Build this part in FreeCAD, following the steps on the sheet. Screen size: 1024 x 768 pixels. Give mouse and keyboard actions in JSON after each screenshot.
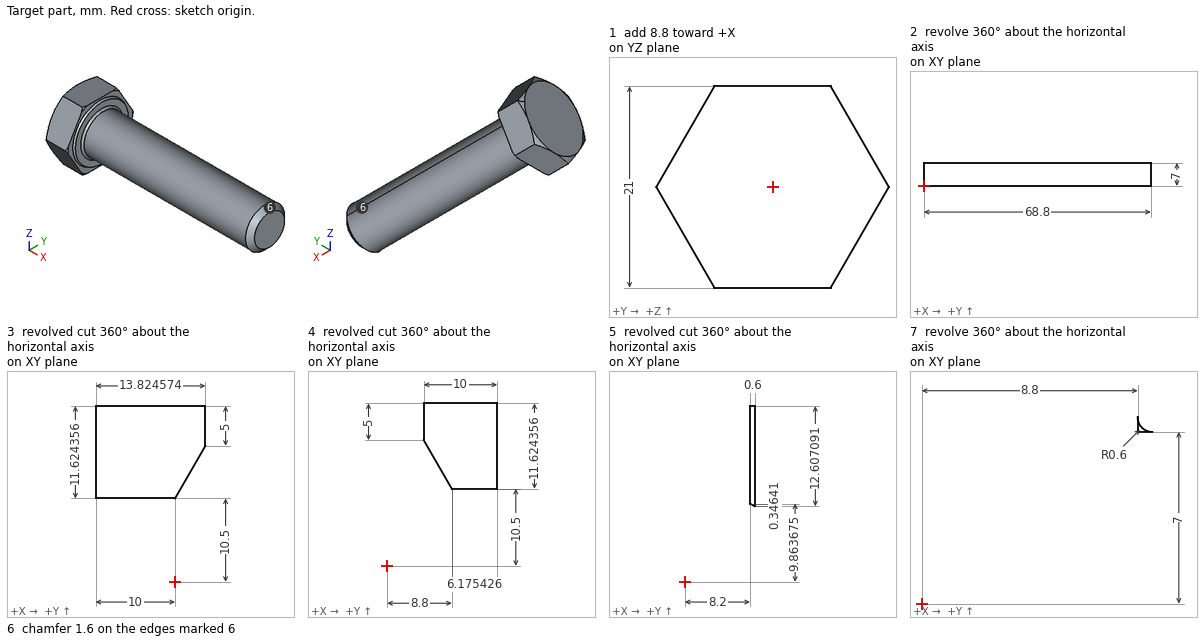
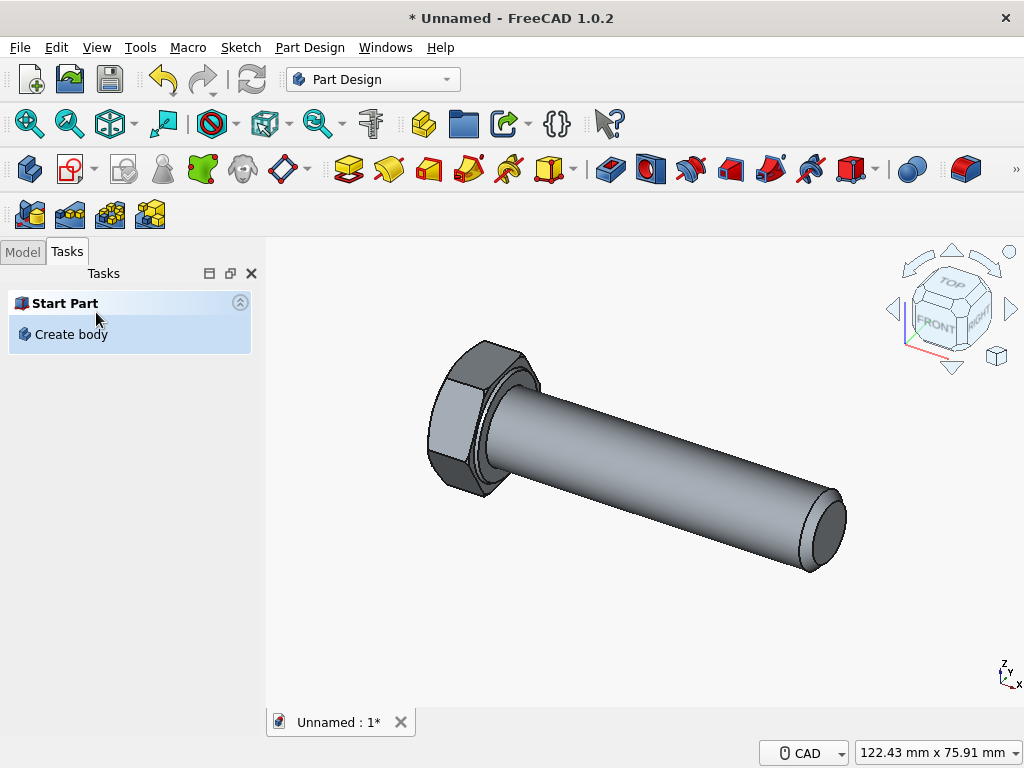
{"action": "left_click", "coordinate": [70, 170]}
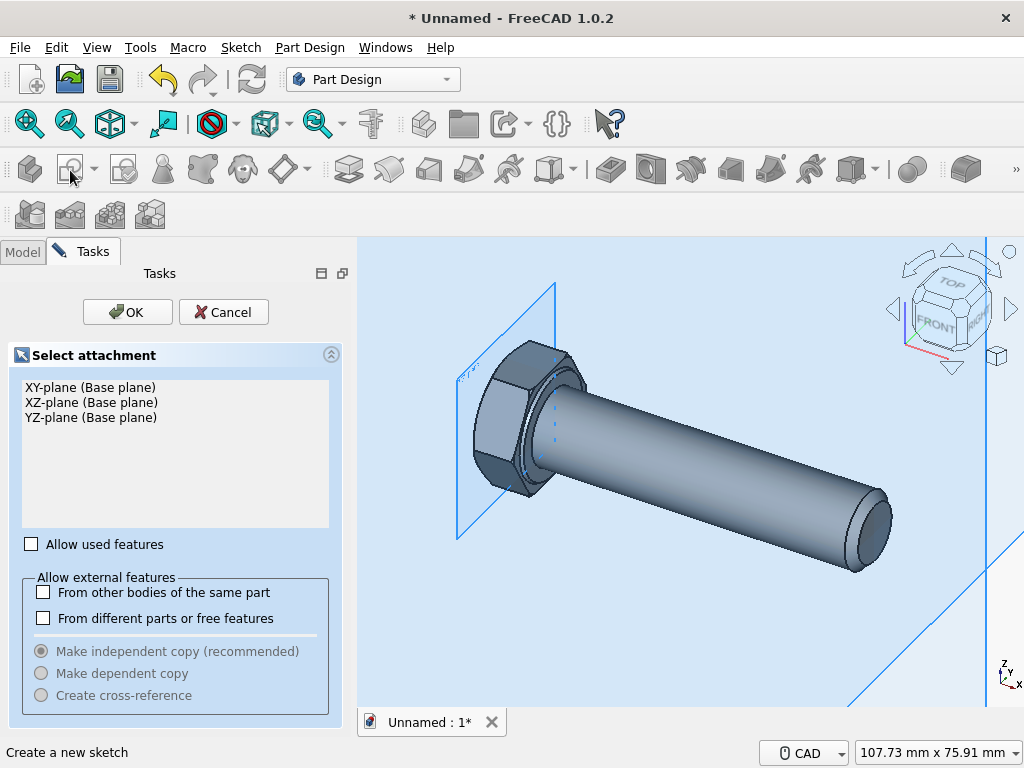
{"action": "left_click", "coordinate": [82, 388]}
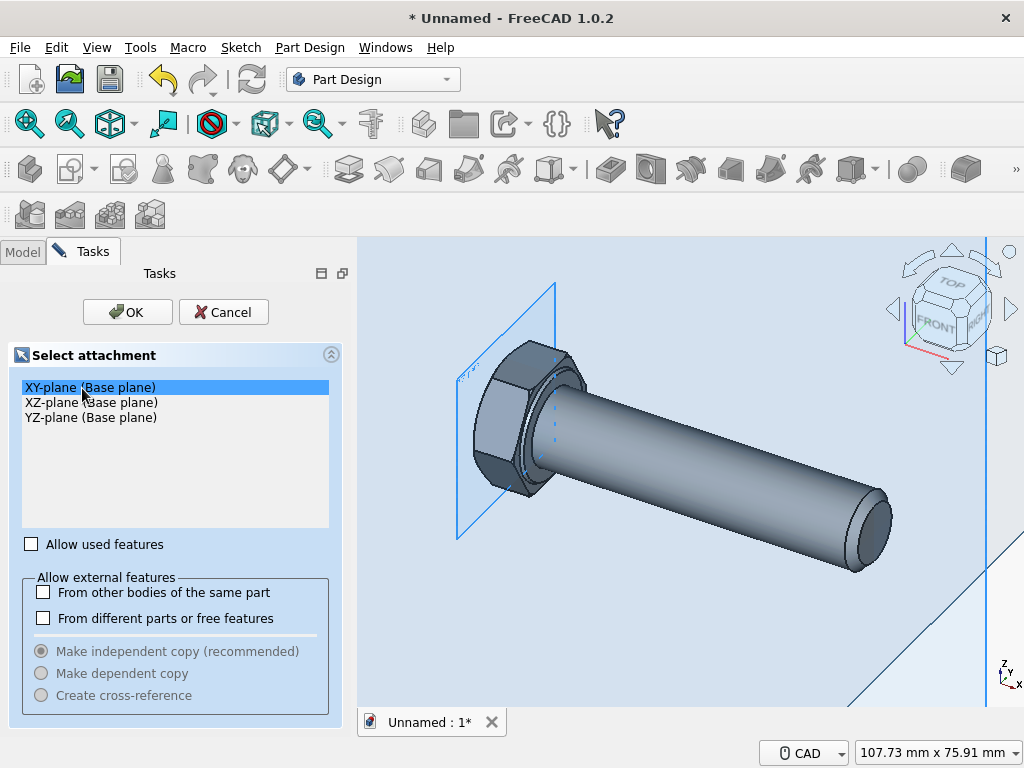
{"action": "left_click", "coordinate": [128, 312]}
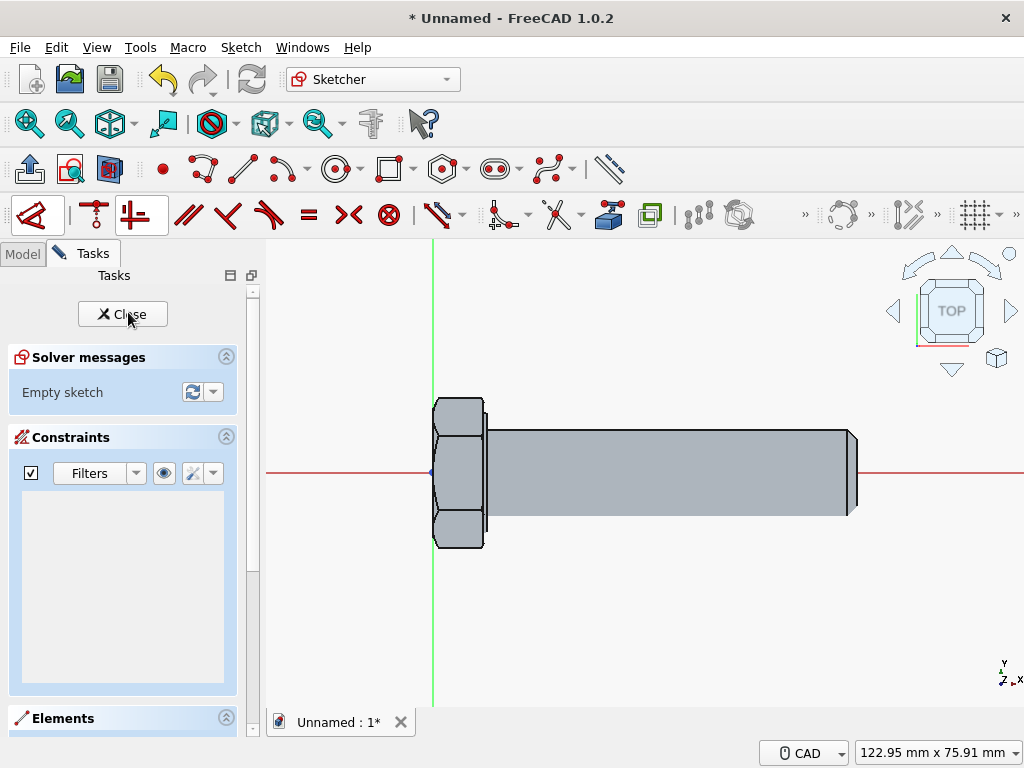
{"action": "left_click", "coordinate": [110, 170]}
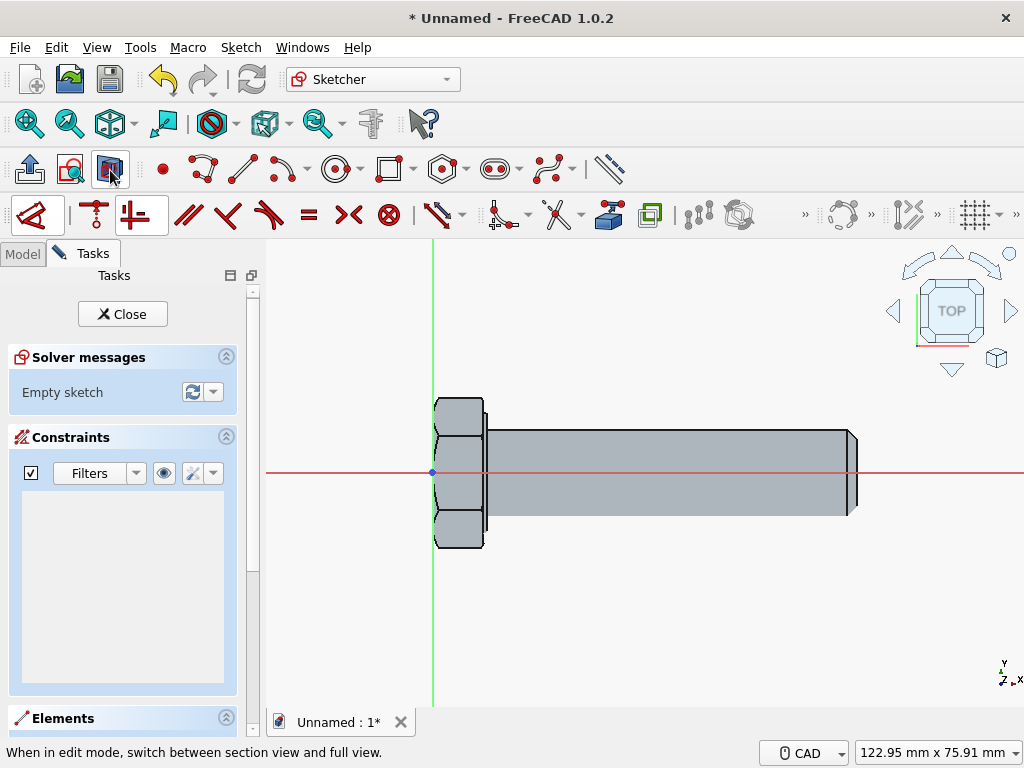
{"action": "scroll", "coordinate": [484, 426], "scroll_direction": "up", "scroll_amount": 15}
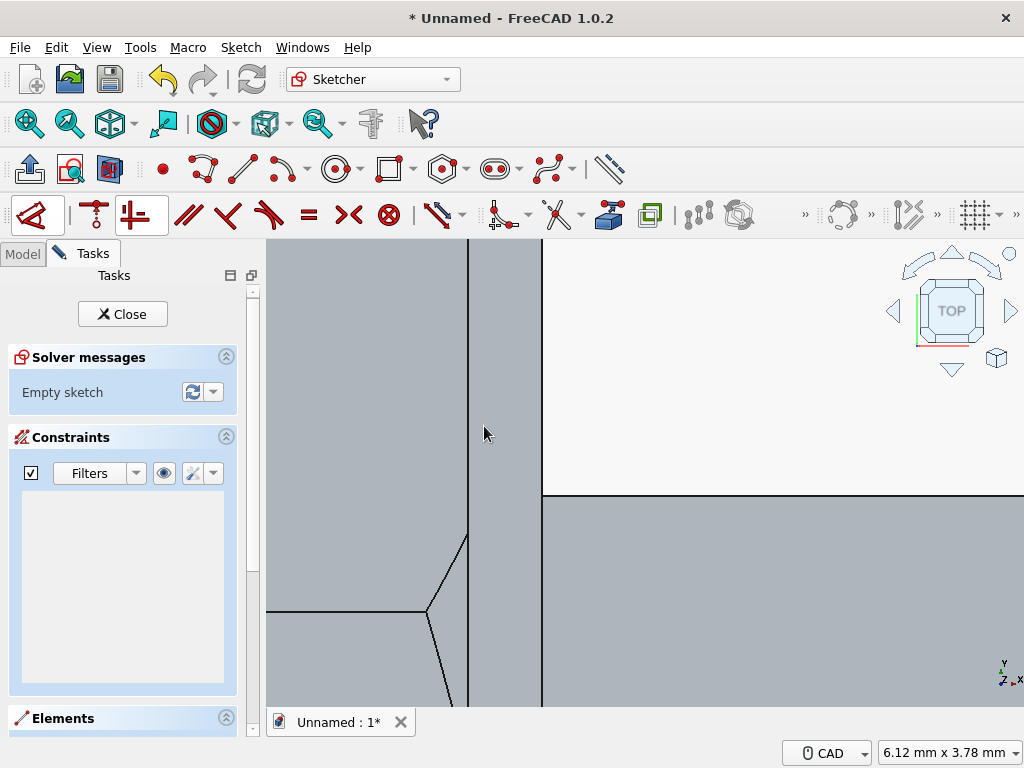
{"action": "scroll", "coordinate": [580, 454], "scroll_direction": "up", "scroll_amount": 7}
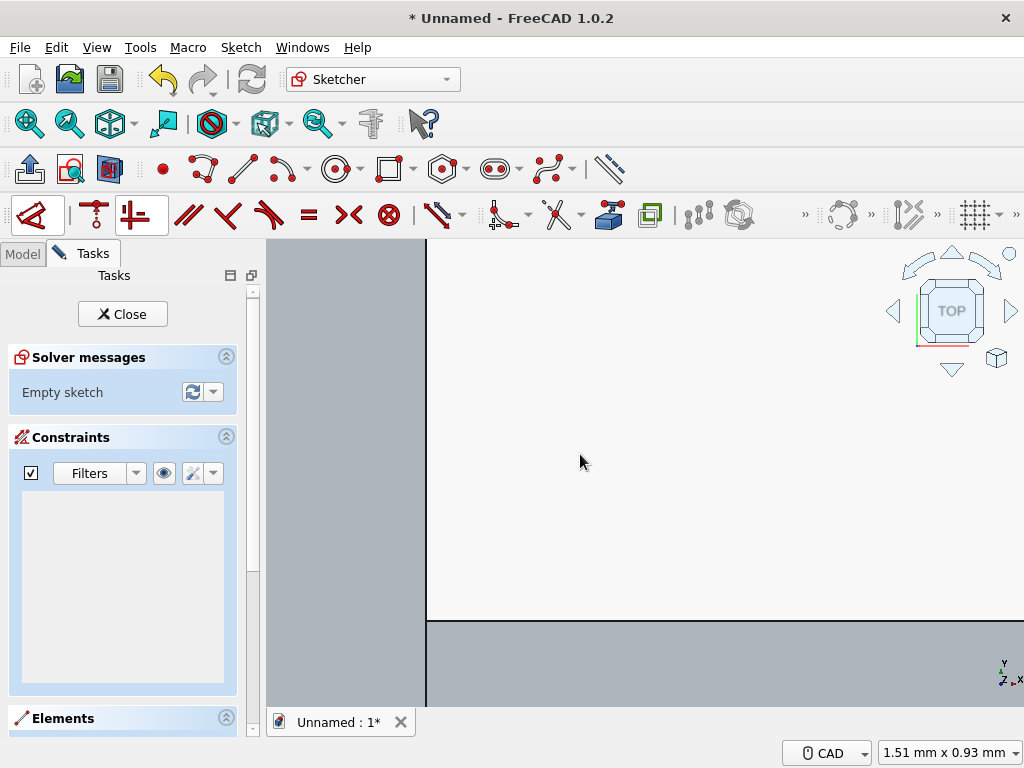
{"action": "key", "text": "g m"}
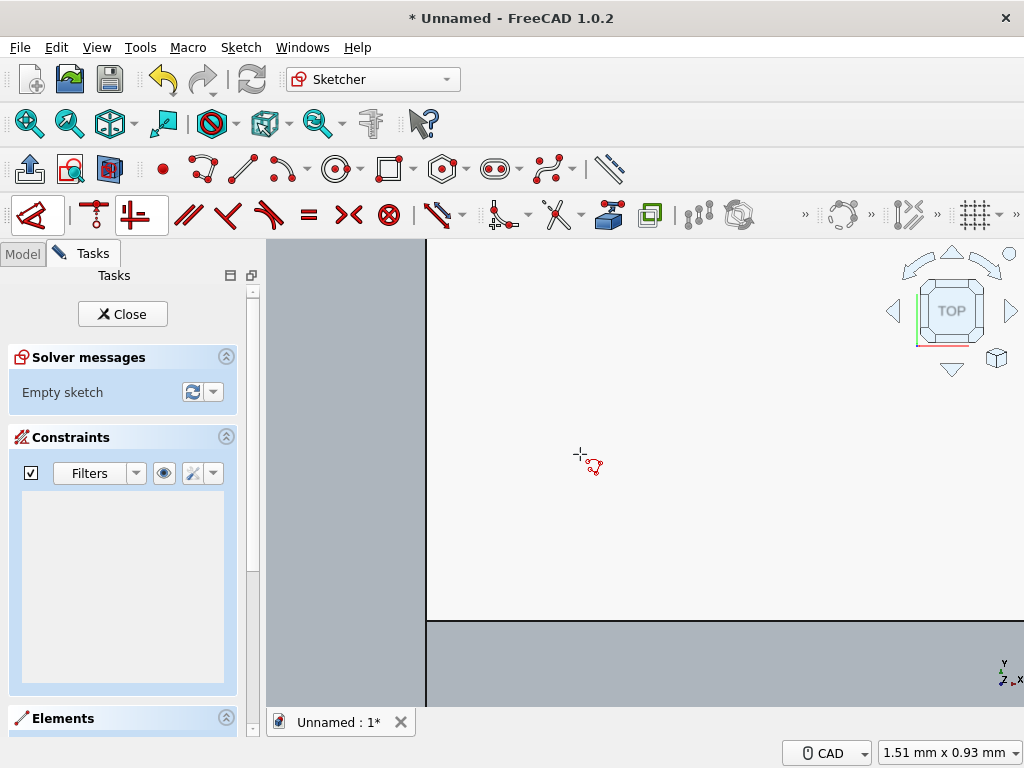
{"action": "left_click", "coordinate": [426, 320]}
{"action": "left_click", "coordinate": [426, 621]}
{"action": "left_click", "coordinate": [727, 621]}
{"action": "right_click", "coordinate": [727, 621]}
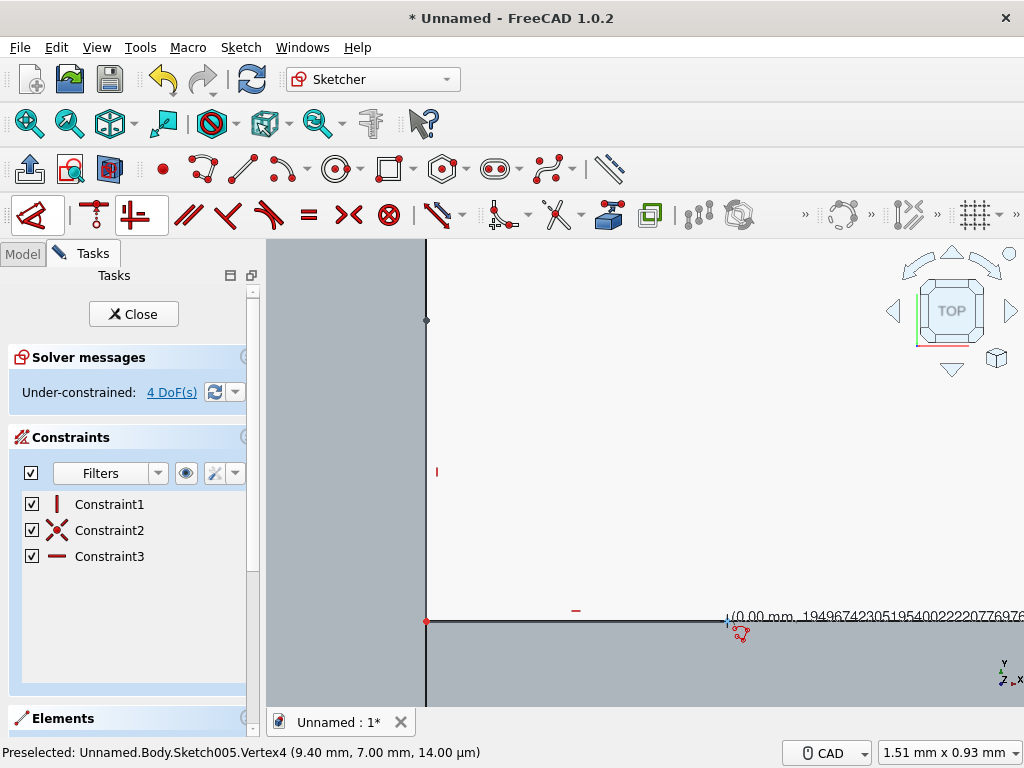
{"action": "left_click", "coordinate": [310, 170]}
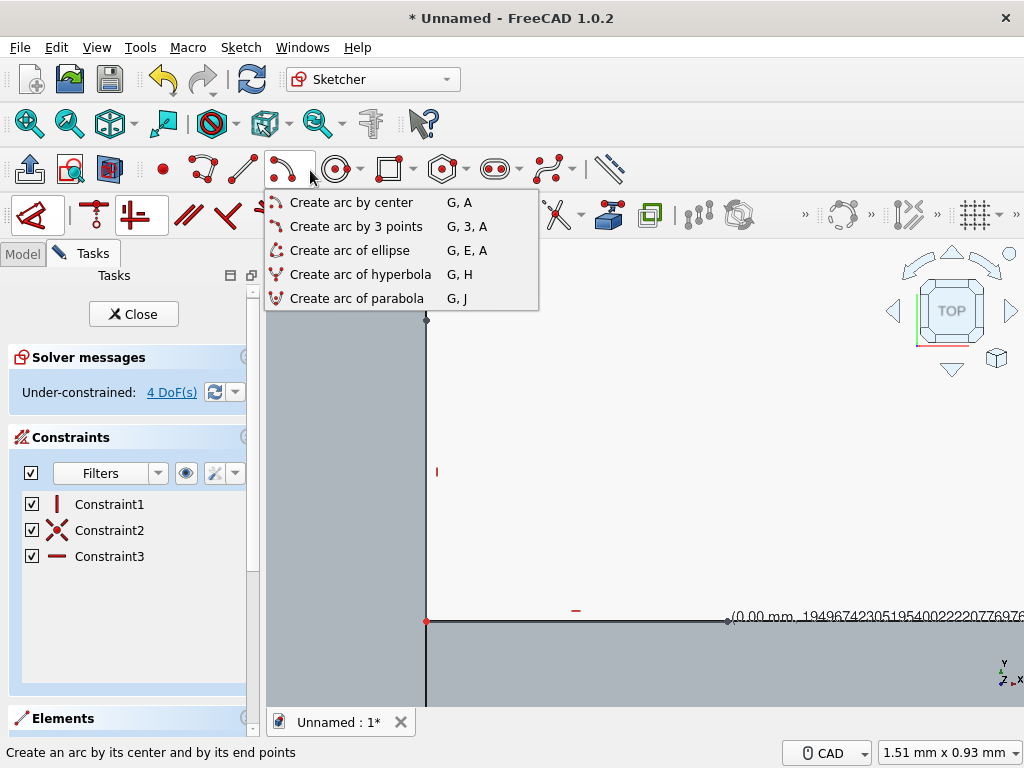
{"action": "left_click", "coordinate": [402, 226]}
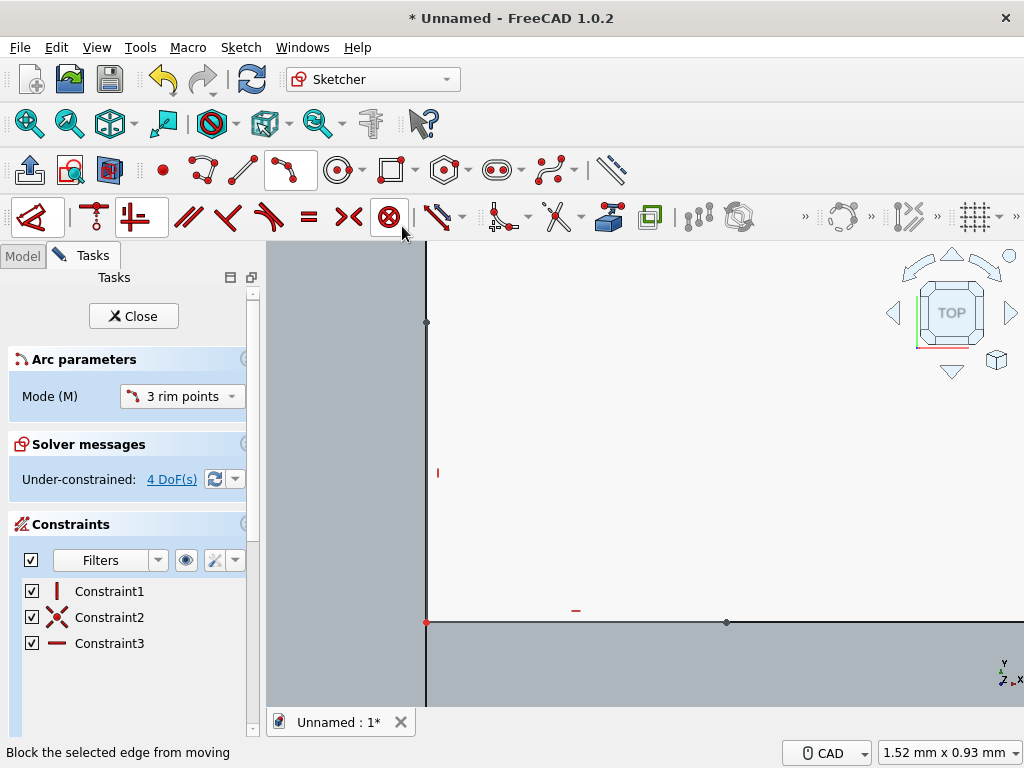
{"action": "left_click", "coordinate": [727, 622]}
{"action": "left_click", "coordinate": [427, 323]}
{"action": "left_click", "coordinate": [514, 534]}
{"action": "key", "text": "Escape"}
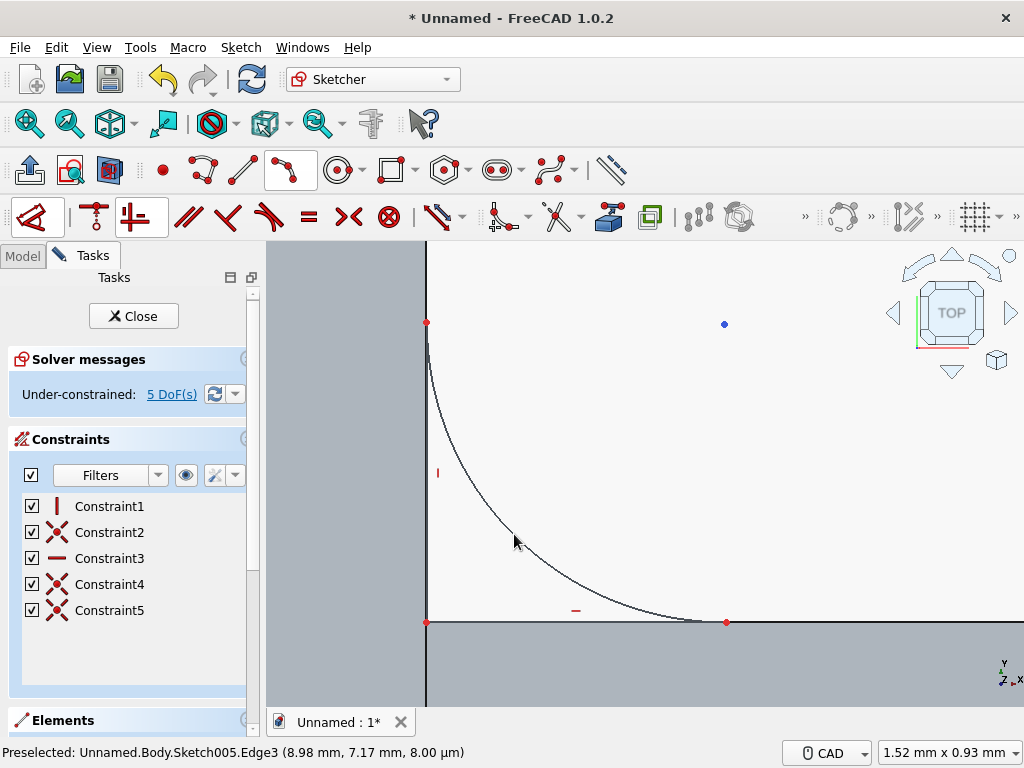
{"action": "left_click", "coordinate": [427, 413]}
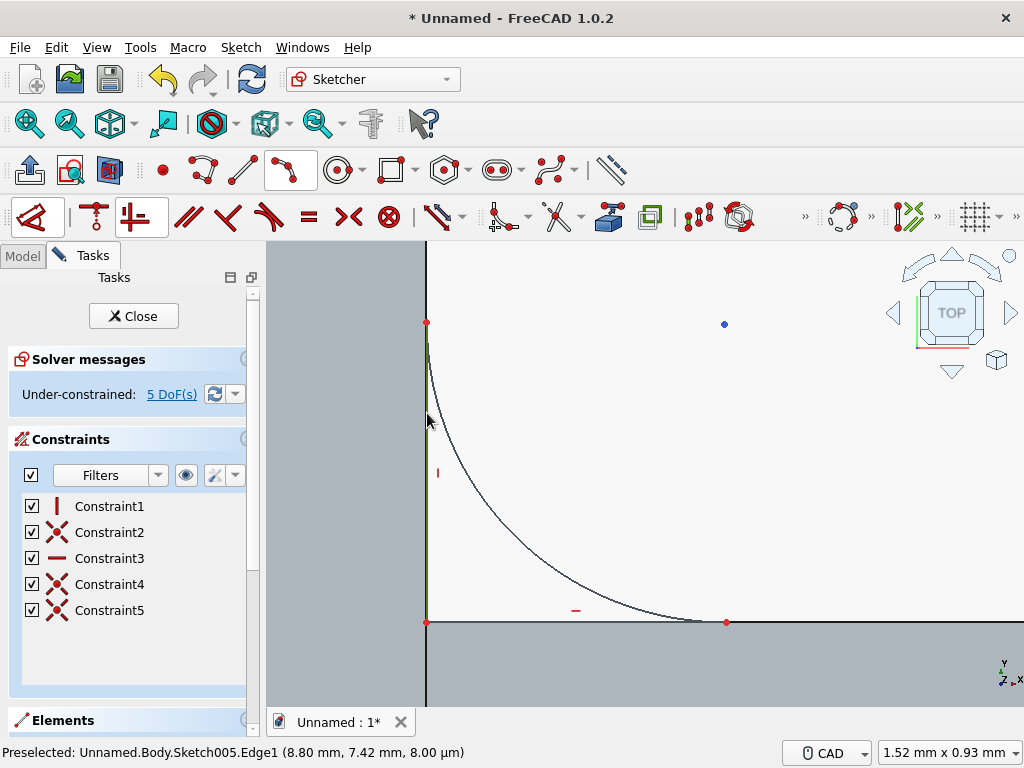
{"action": "left_click", "coordinate": [459, 459]}